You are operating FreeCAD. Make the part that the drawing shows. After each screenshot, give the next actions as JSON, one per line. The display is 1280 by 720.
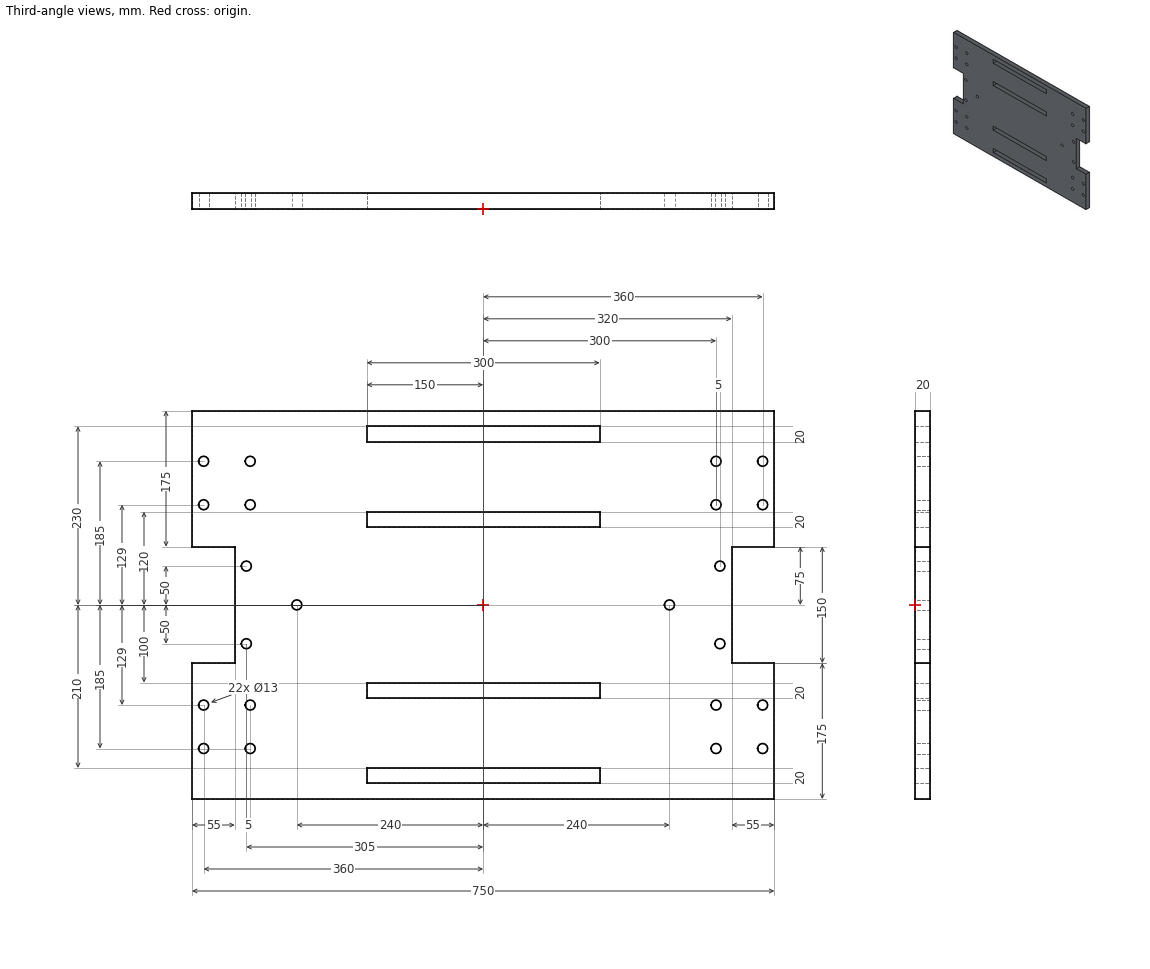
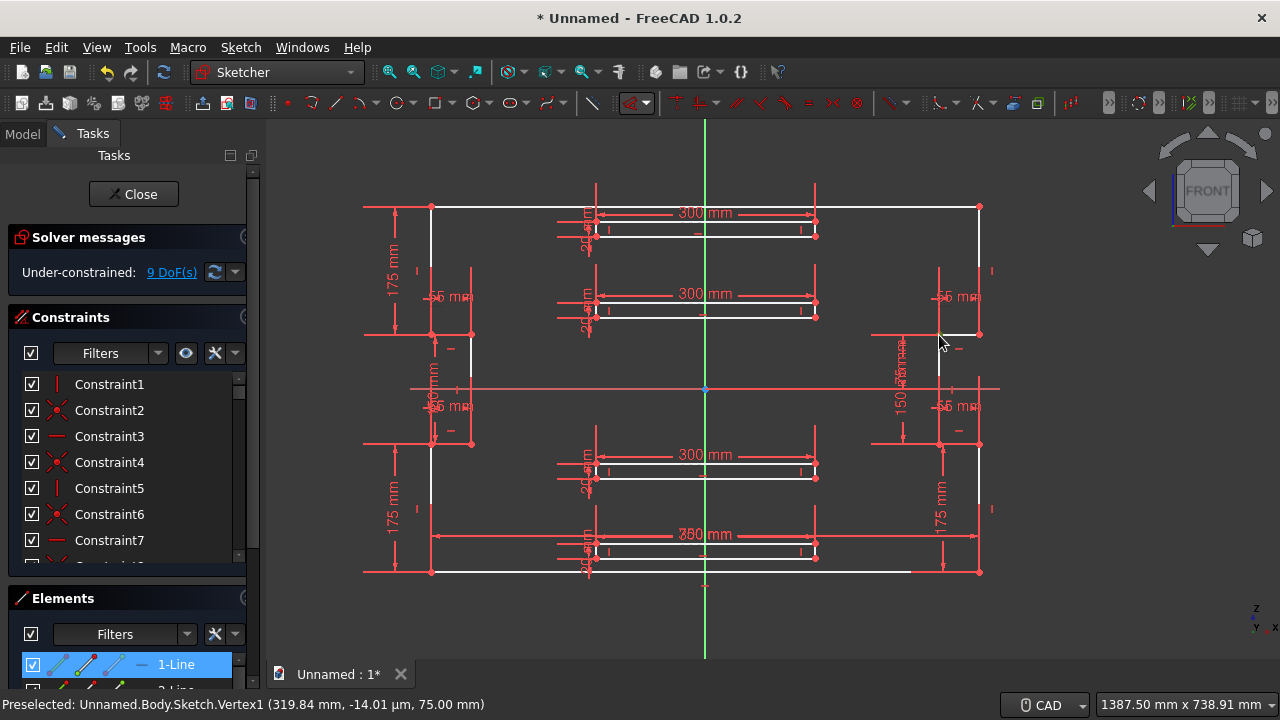
{"action": "left_click", "coordinate": [648, 104]}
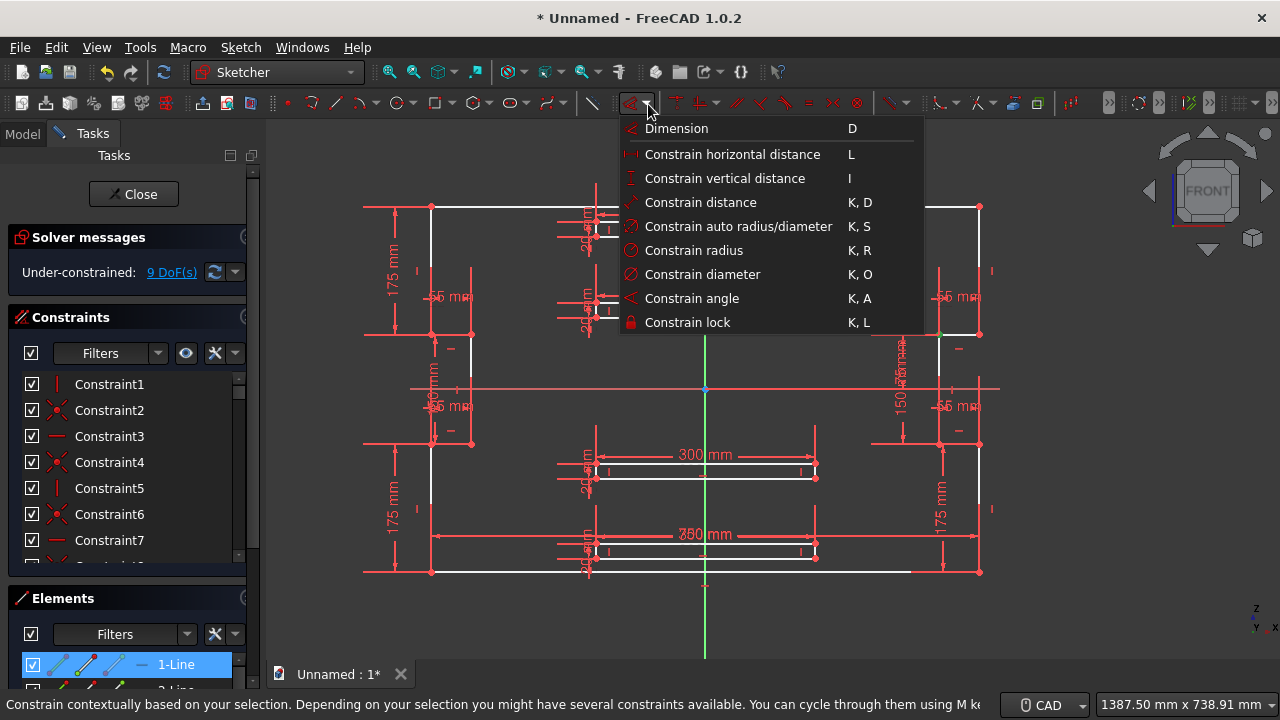
{"action": "left_click", "coordinate": [772, 154]}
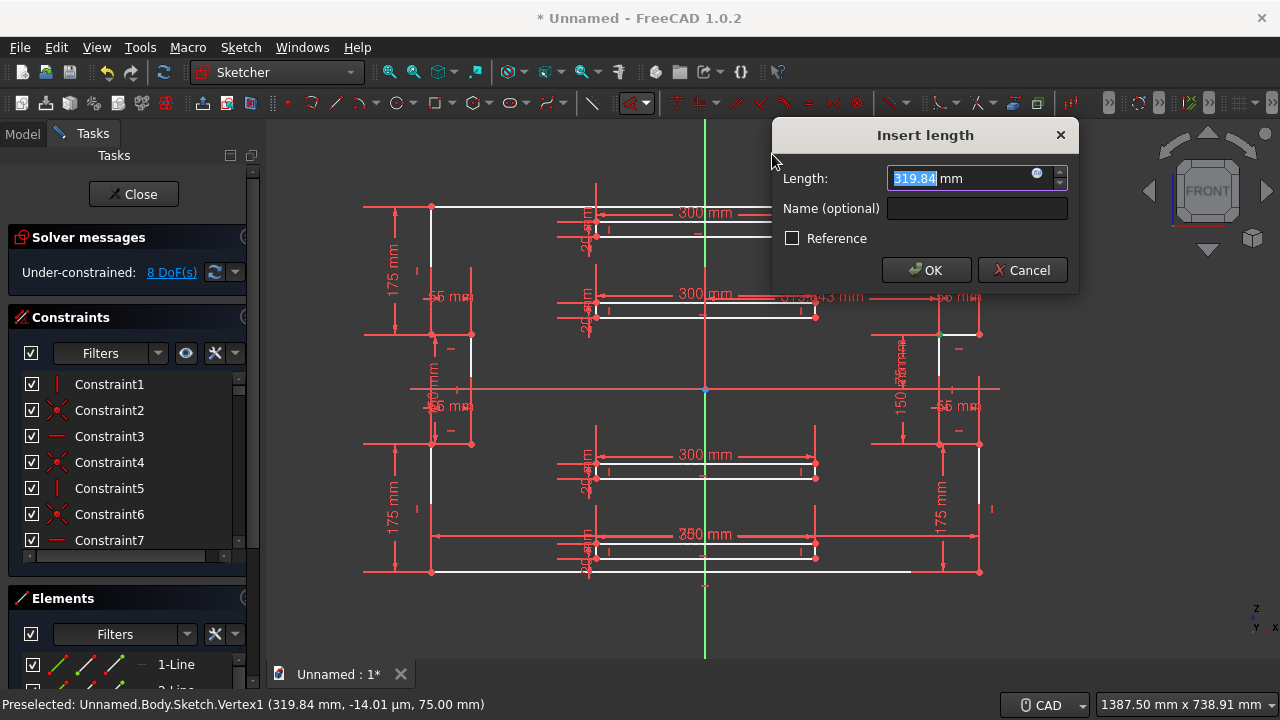
{"action": "type", "text": "320"}
{"action": "key", "text": "Return"}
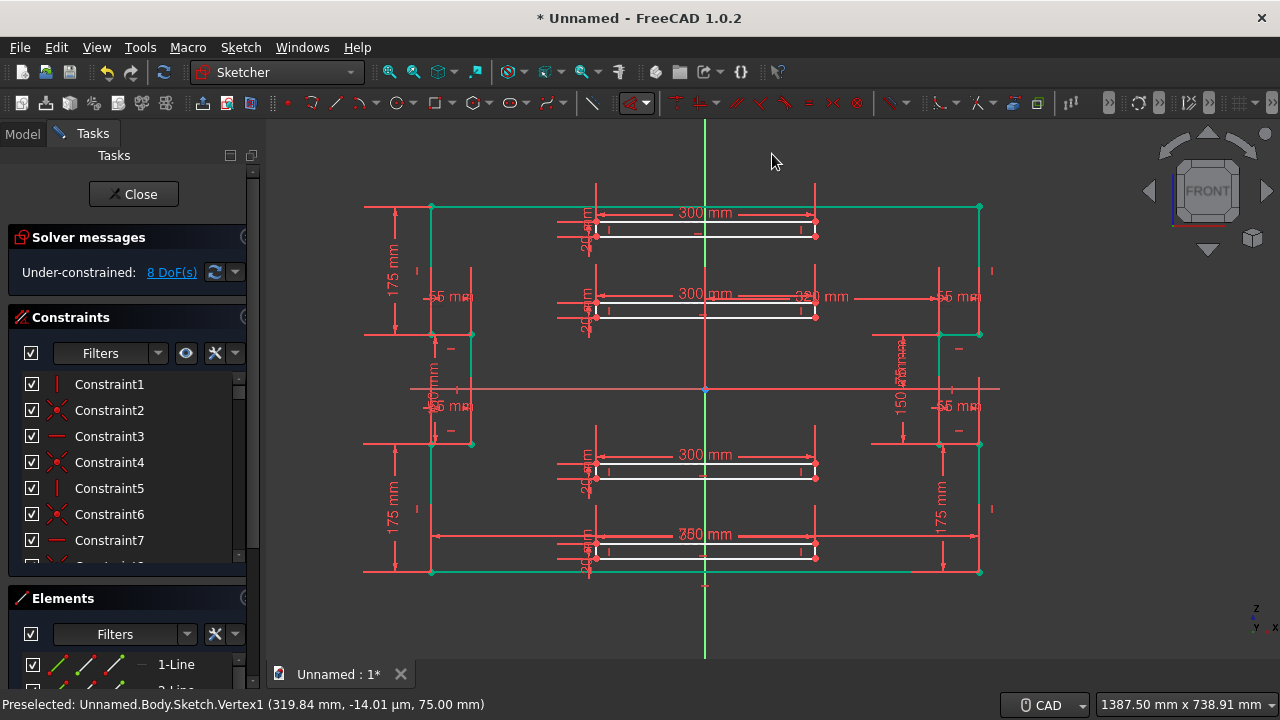
{"action": "left_click", "coordinate": [596, 222]}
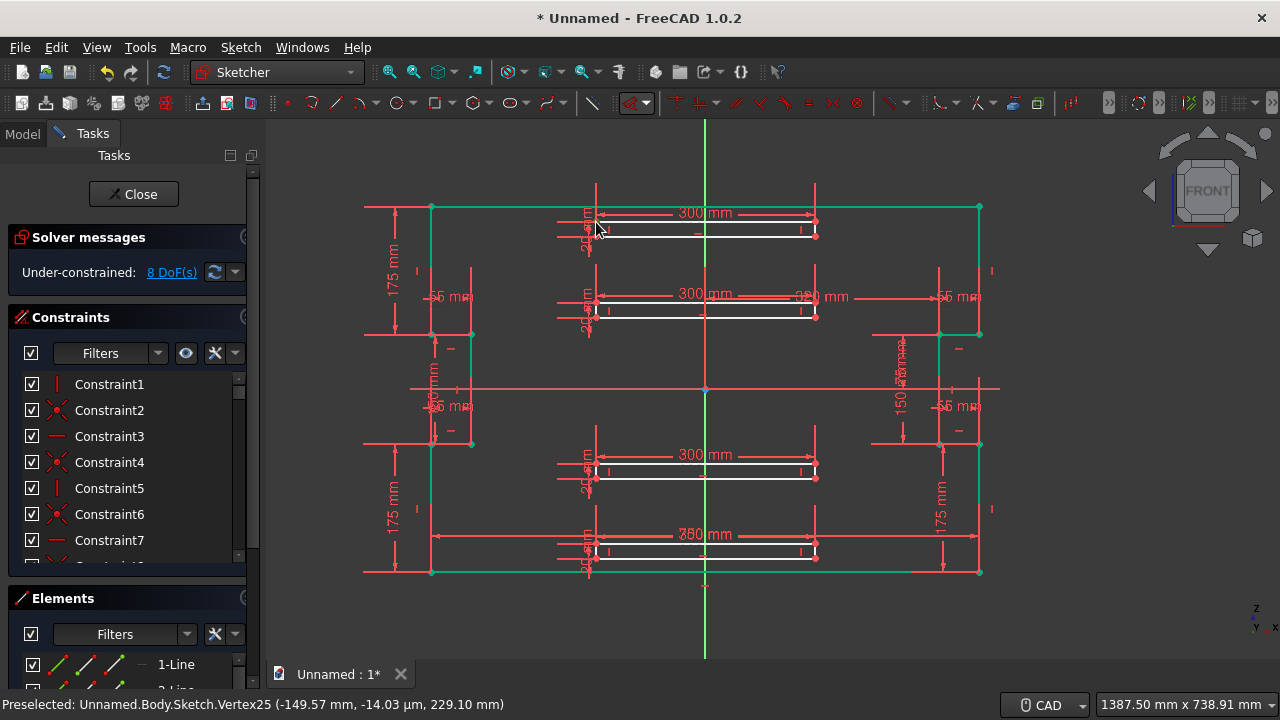
{"action": "left_click", "coordinate": [648, 104]}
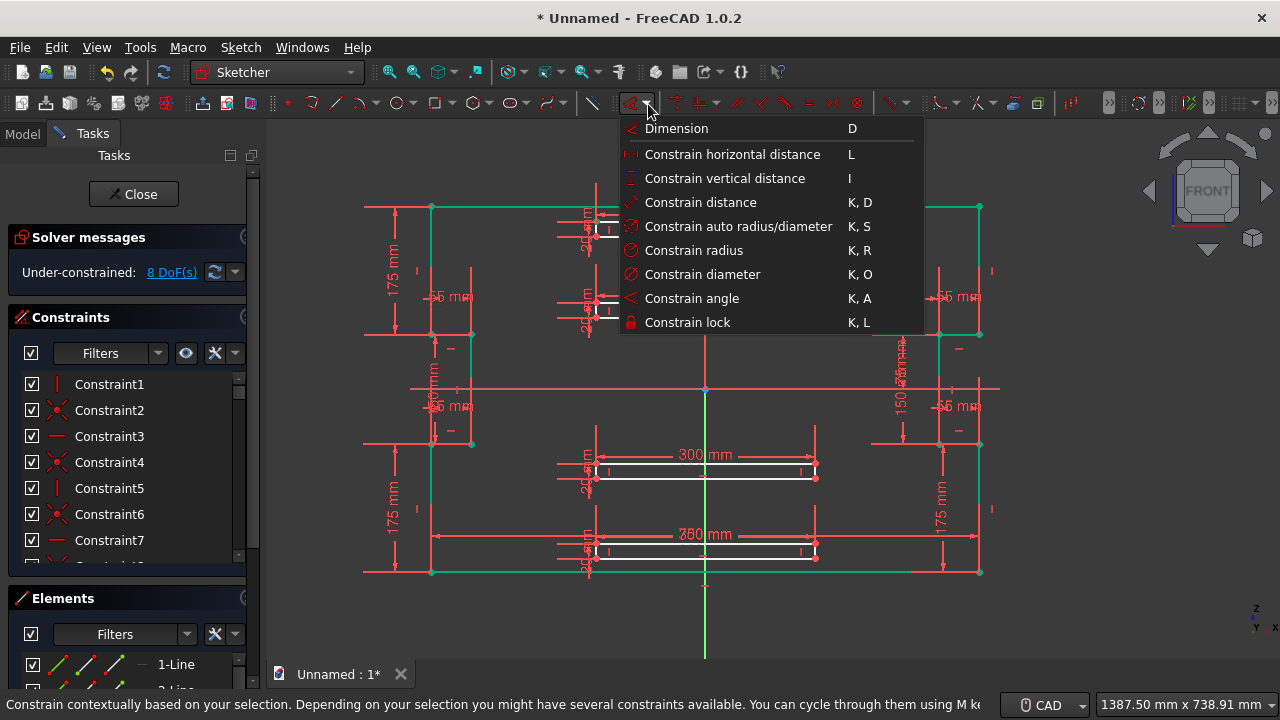
{"action": "left_click", "coordinate": [772, 154]}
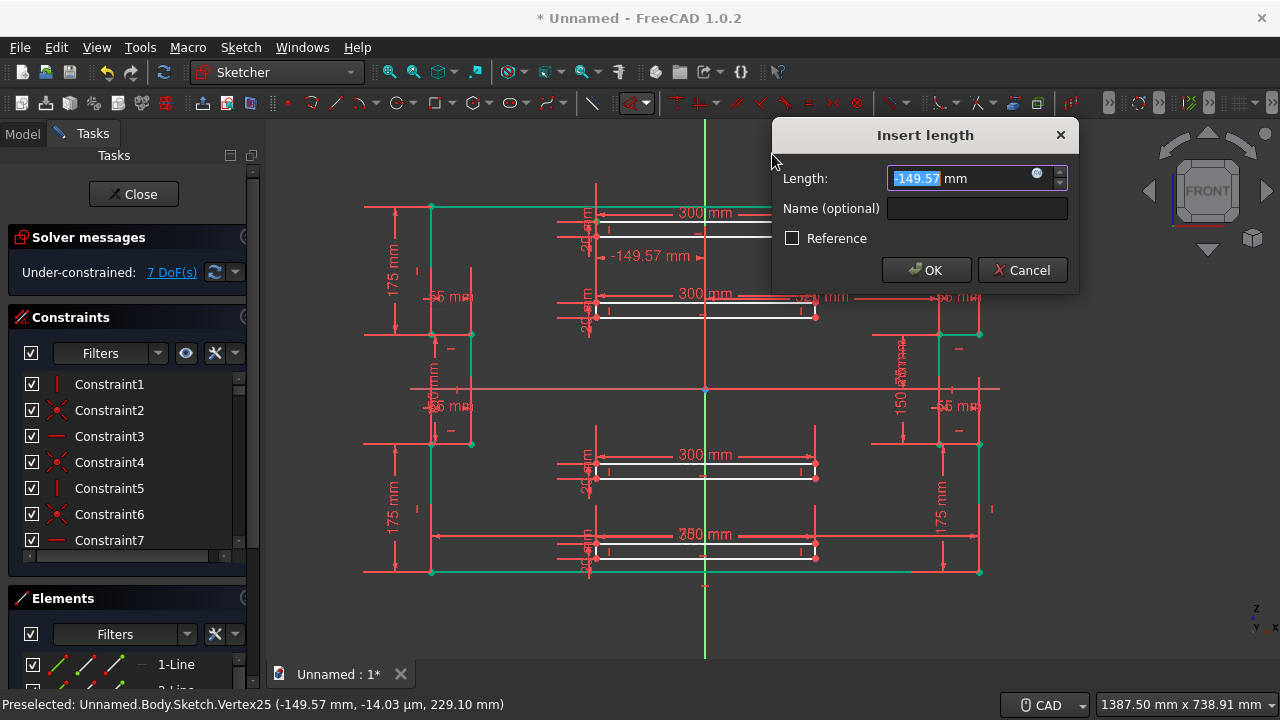
{"action": "type", "text": "-150"}
{"action": "key", "text": "Return"}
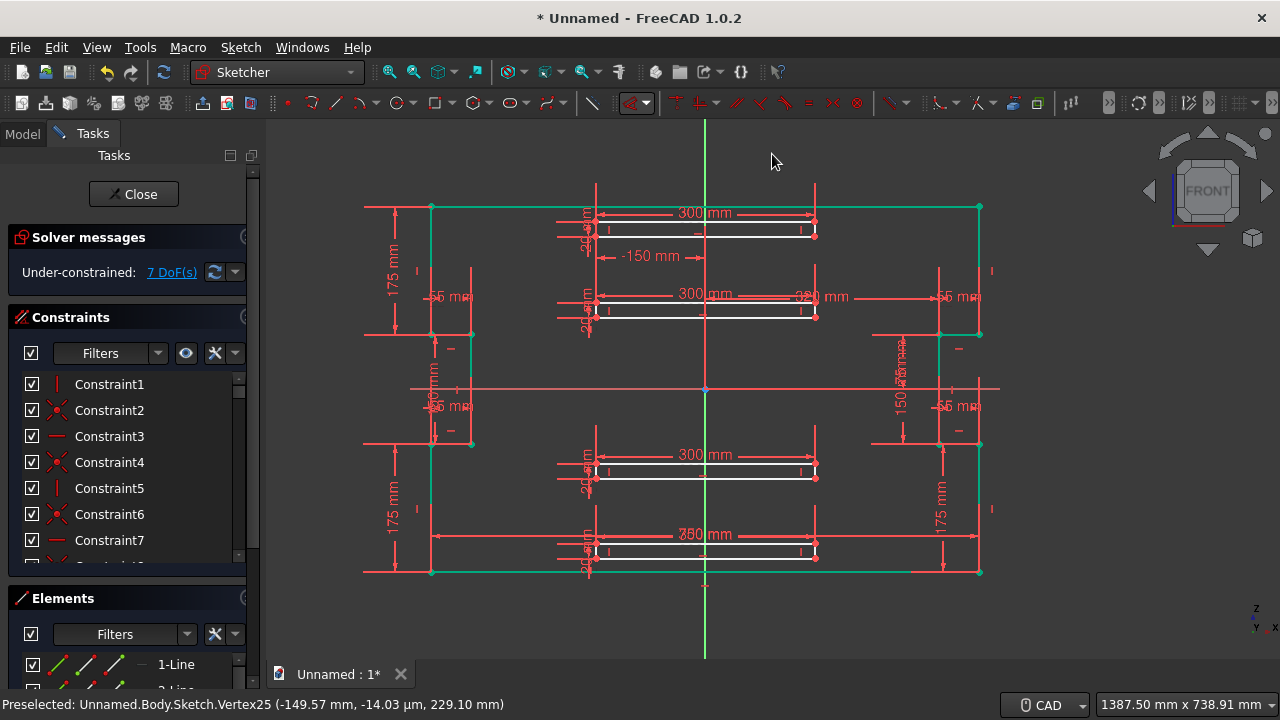
{"action": "left_click", "coordinate": [596, 222]}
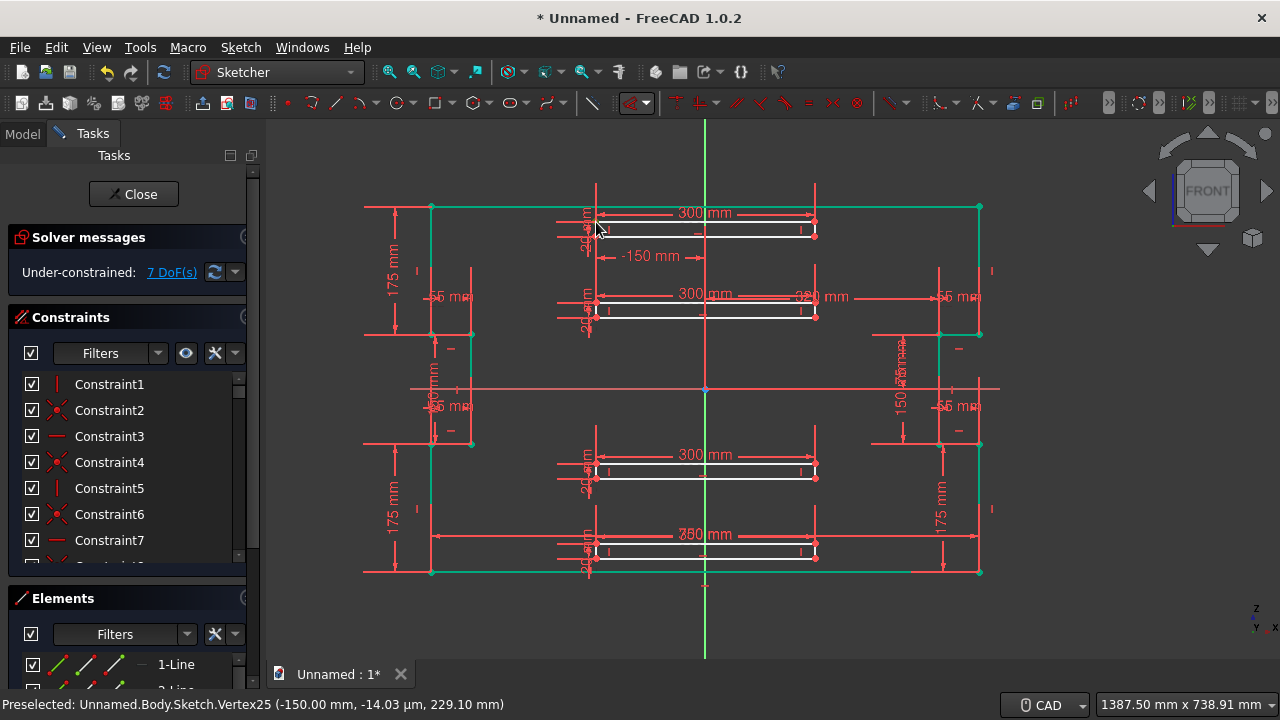
{"action": "left_click", "coordinate": [648, 104]}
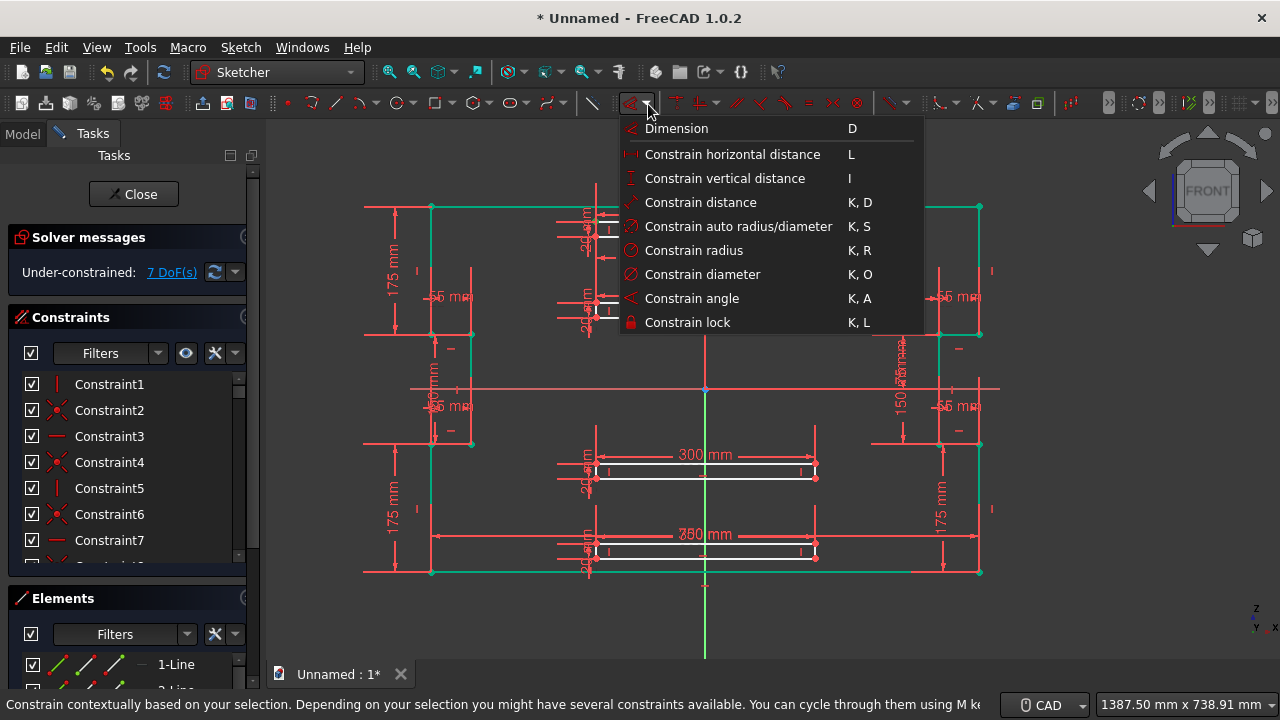
{"action": "left_click", "coordinate": [772, 178]}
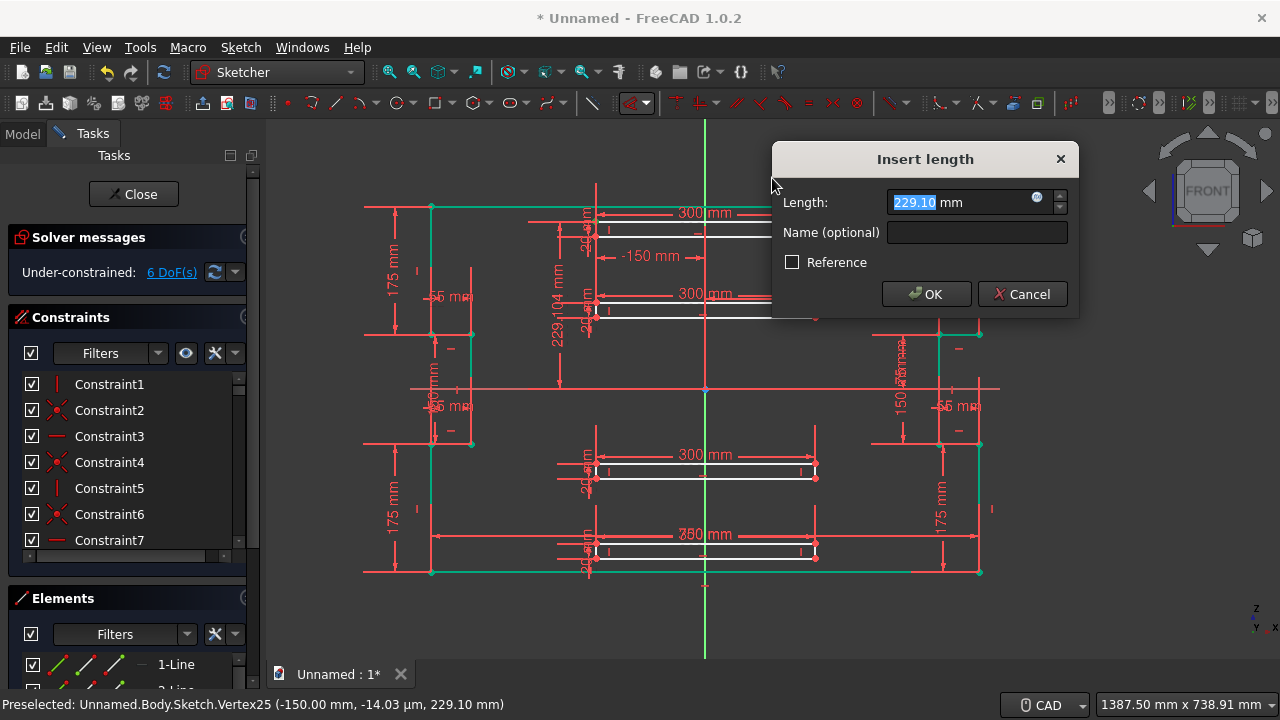
{"action": "type", "text": "230"}
{"action": "key", "text": "Return"}